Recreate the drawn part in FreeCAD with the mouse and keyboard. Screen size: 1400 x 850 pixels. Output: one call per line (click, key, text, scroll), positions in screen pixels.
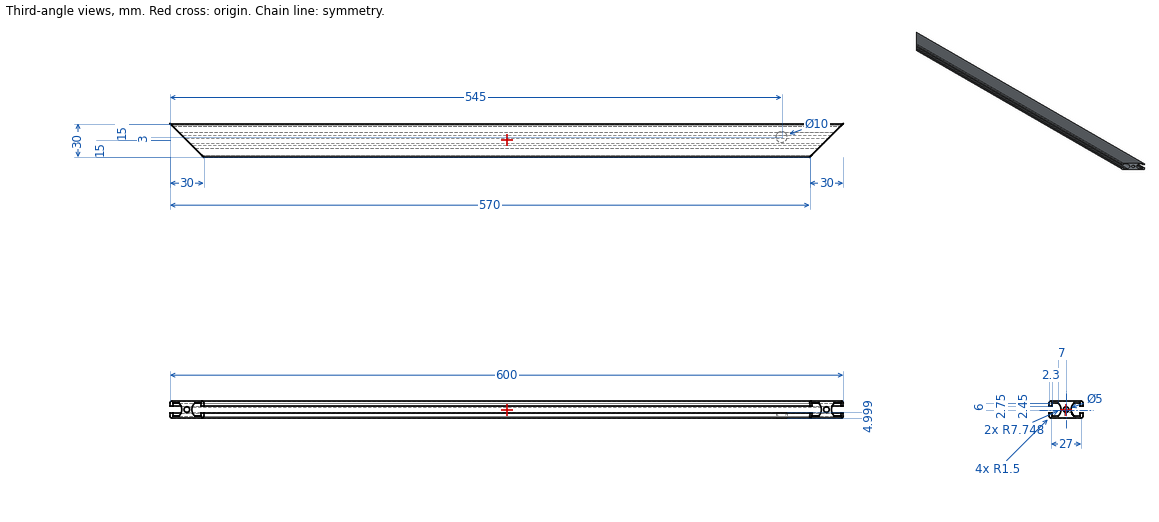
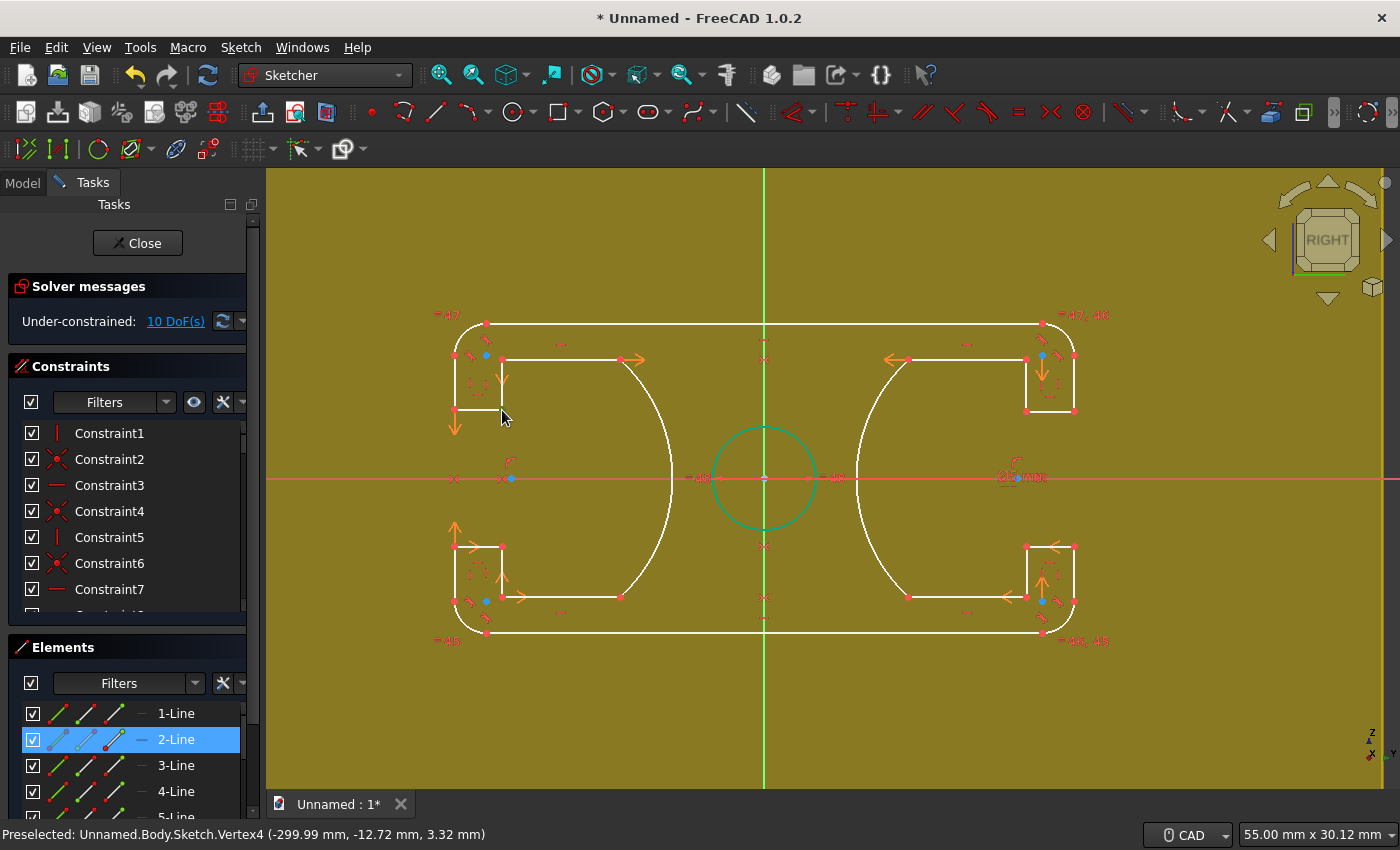
click(1026, 412)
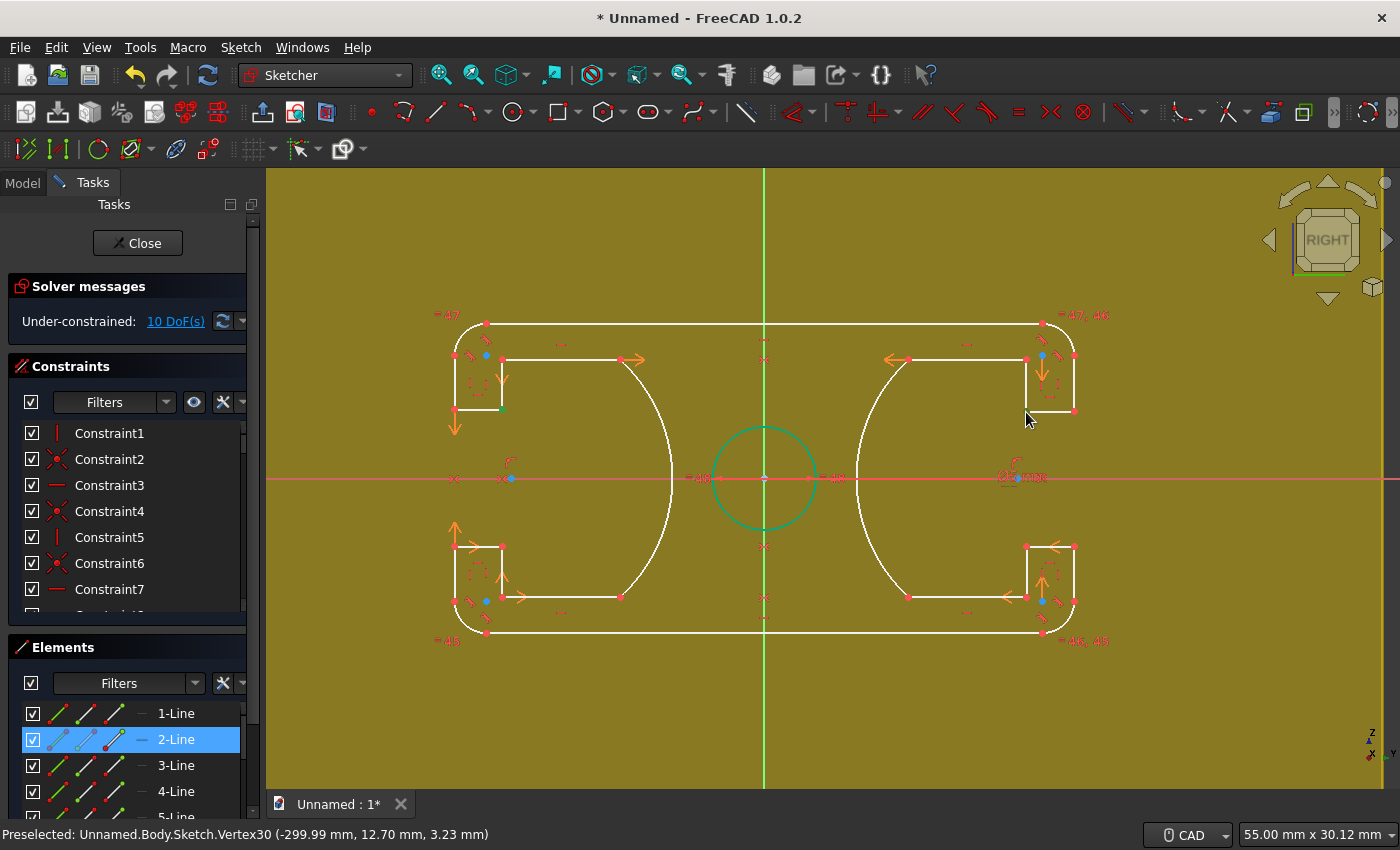
click(764, 721)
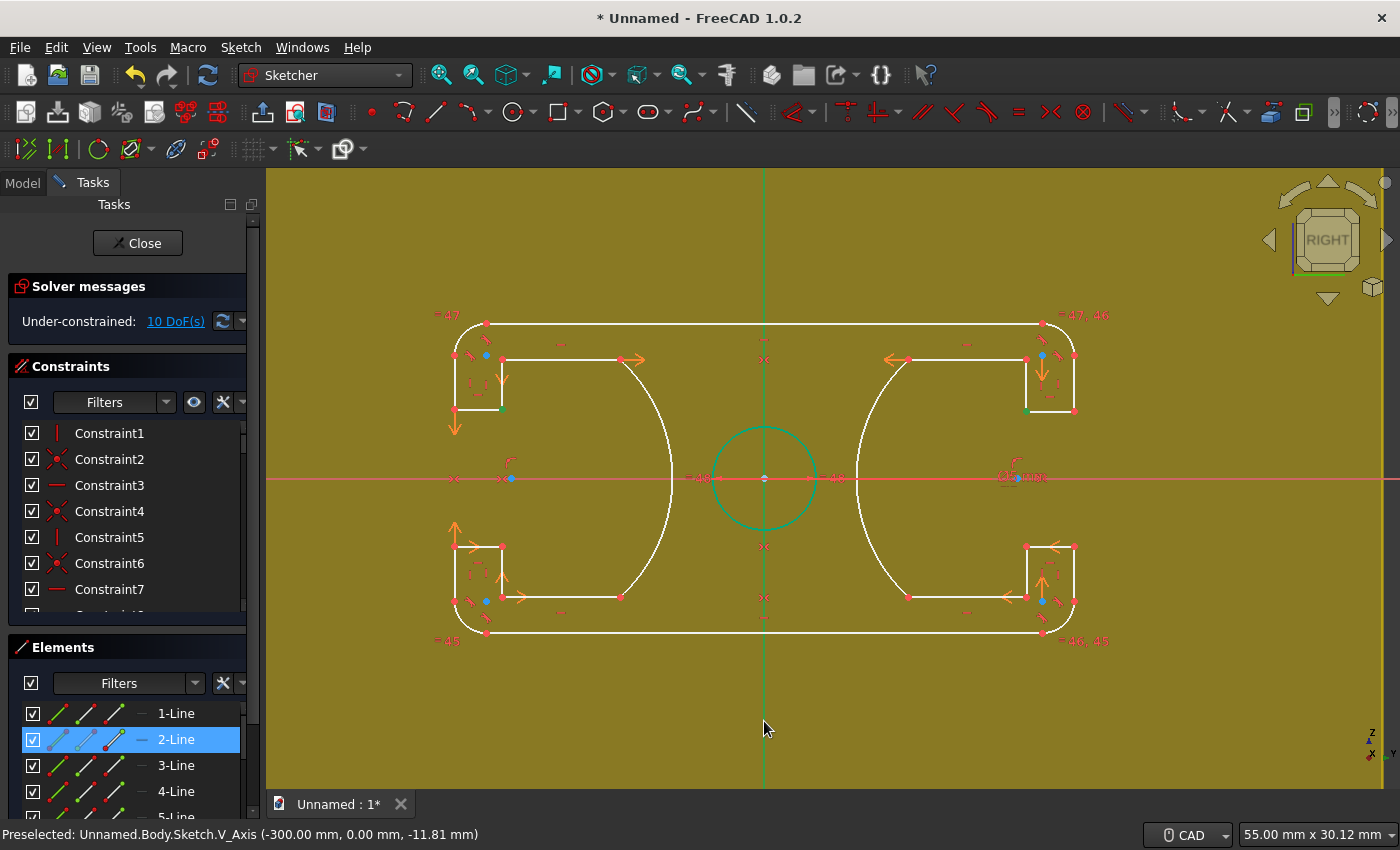
click(1052, 112)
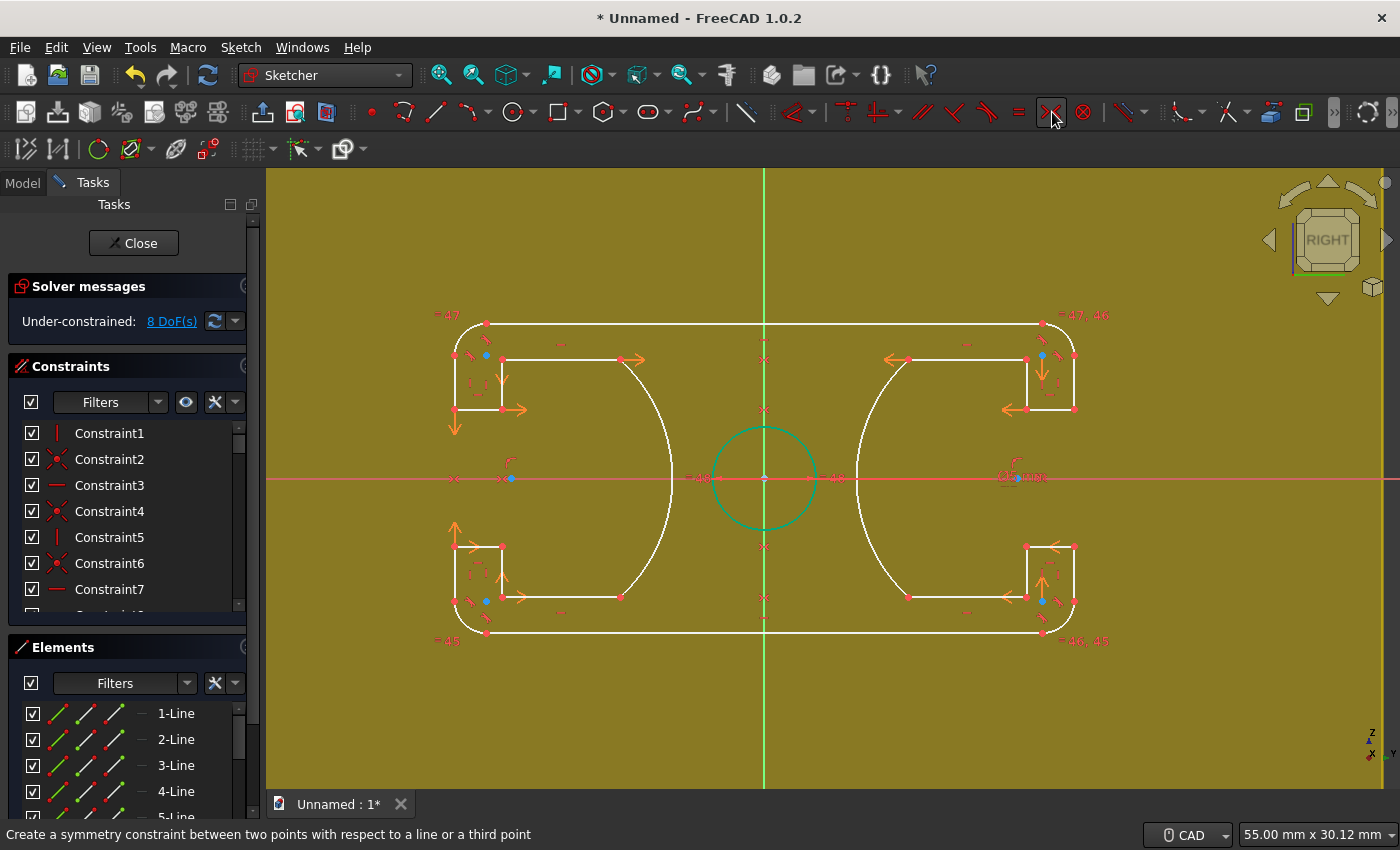
click(792, 112)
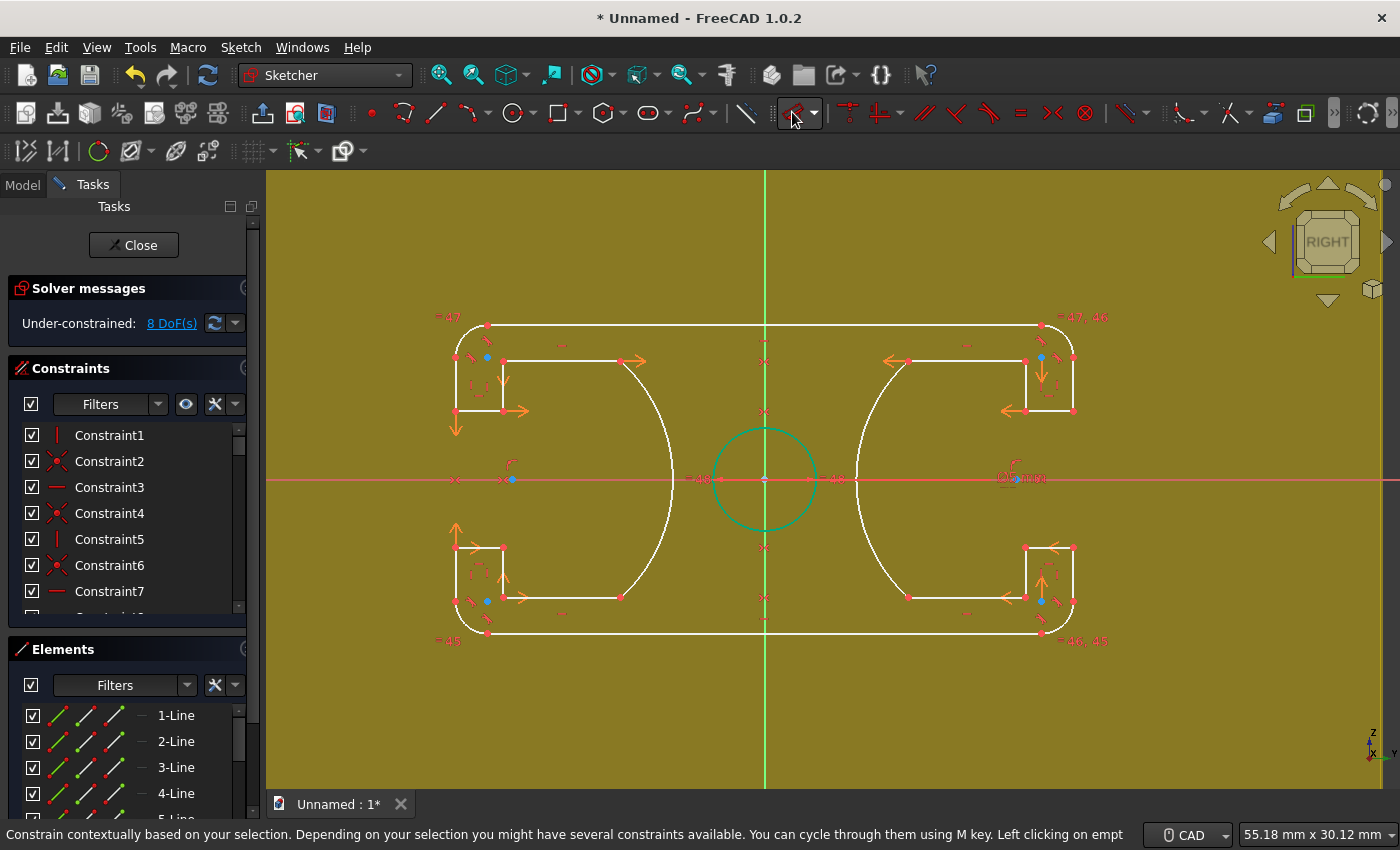
click(664, 532)
click(694, 542)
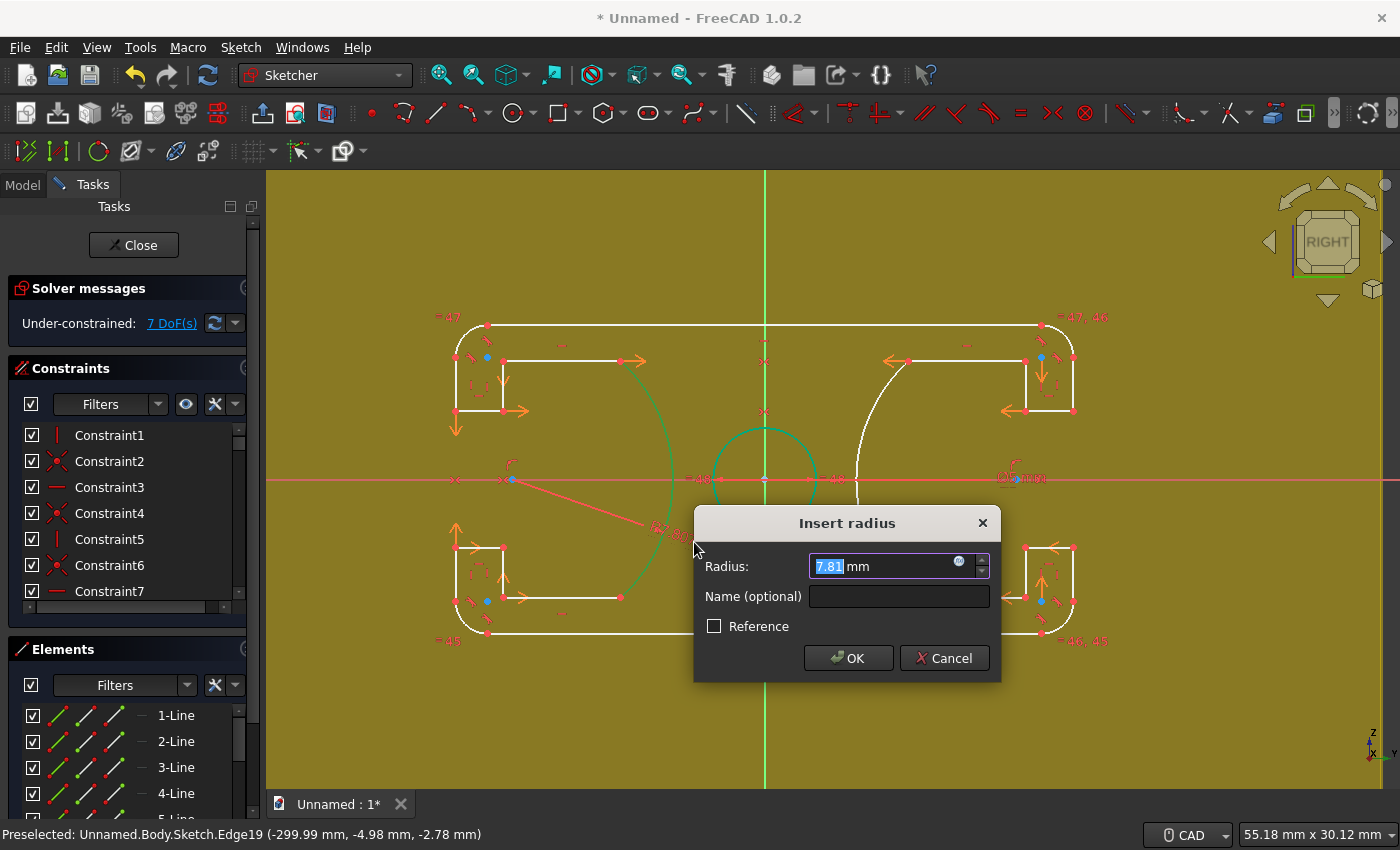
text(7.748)
key(Return)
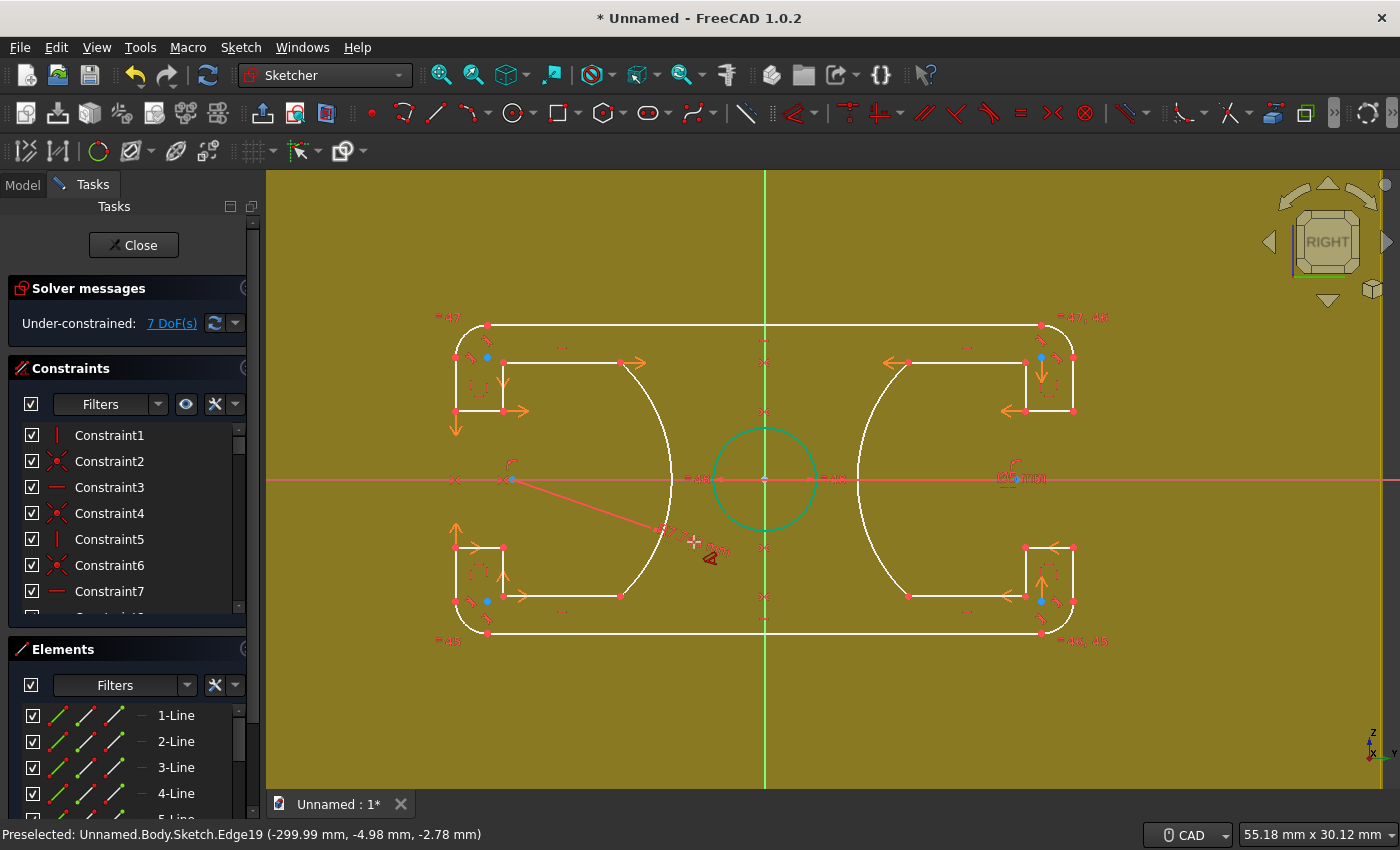
scroll(459, 616, up, 2)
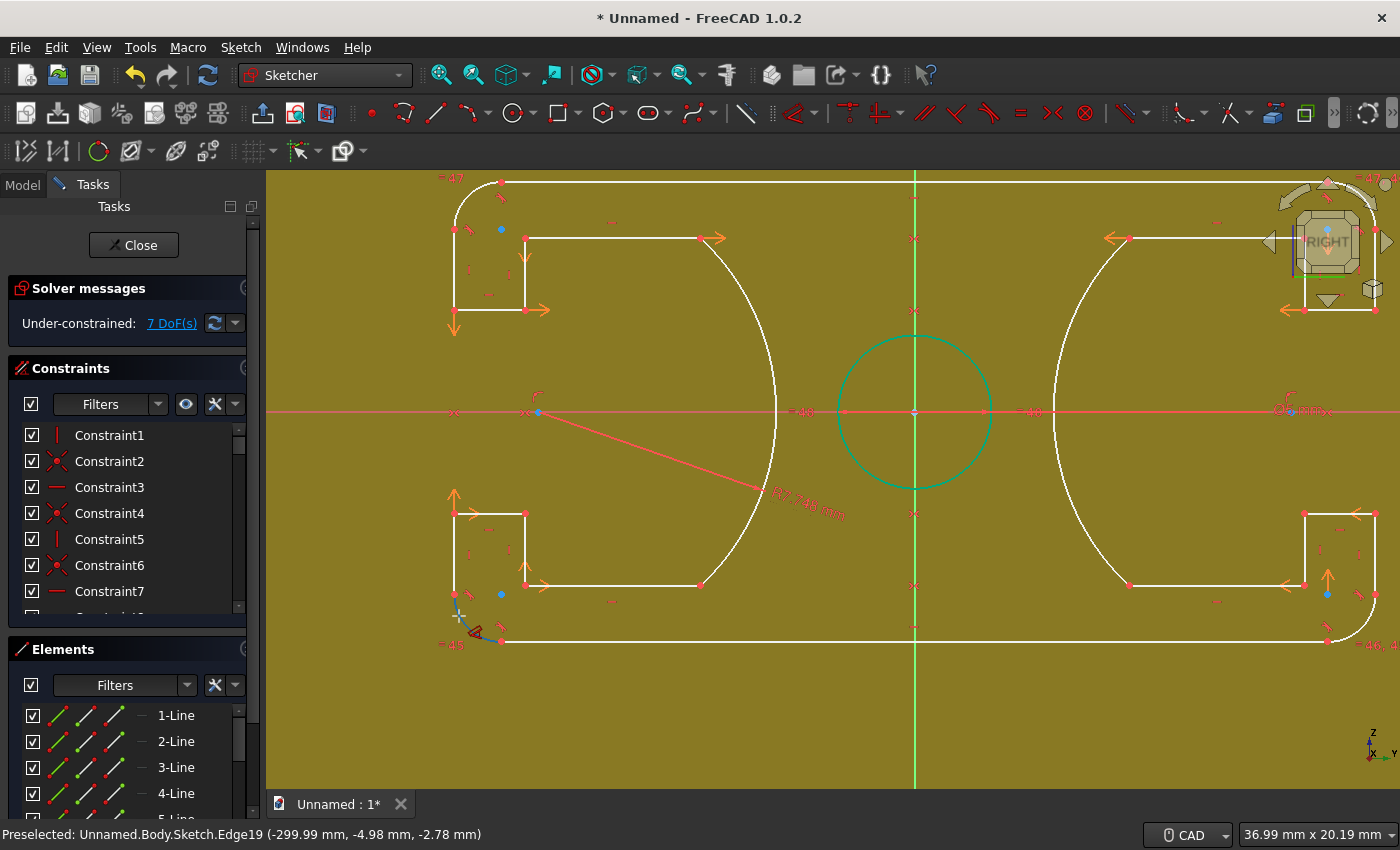
click(460, 616)
click(432, 631)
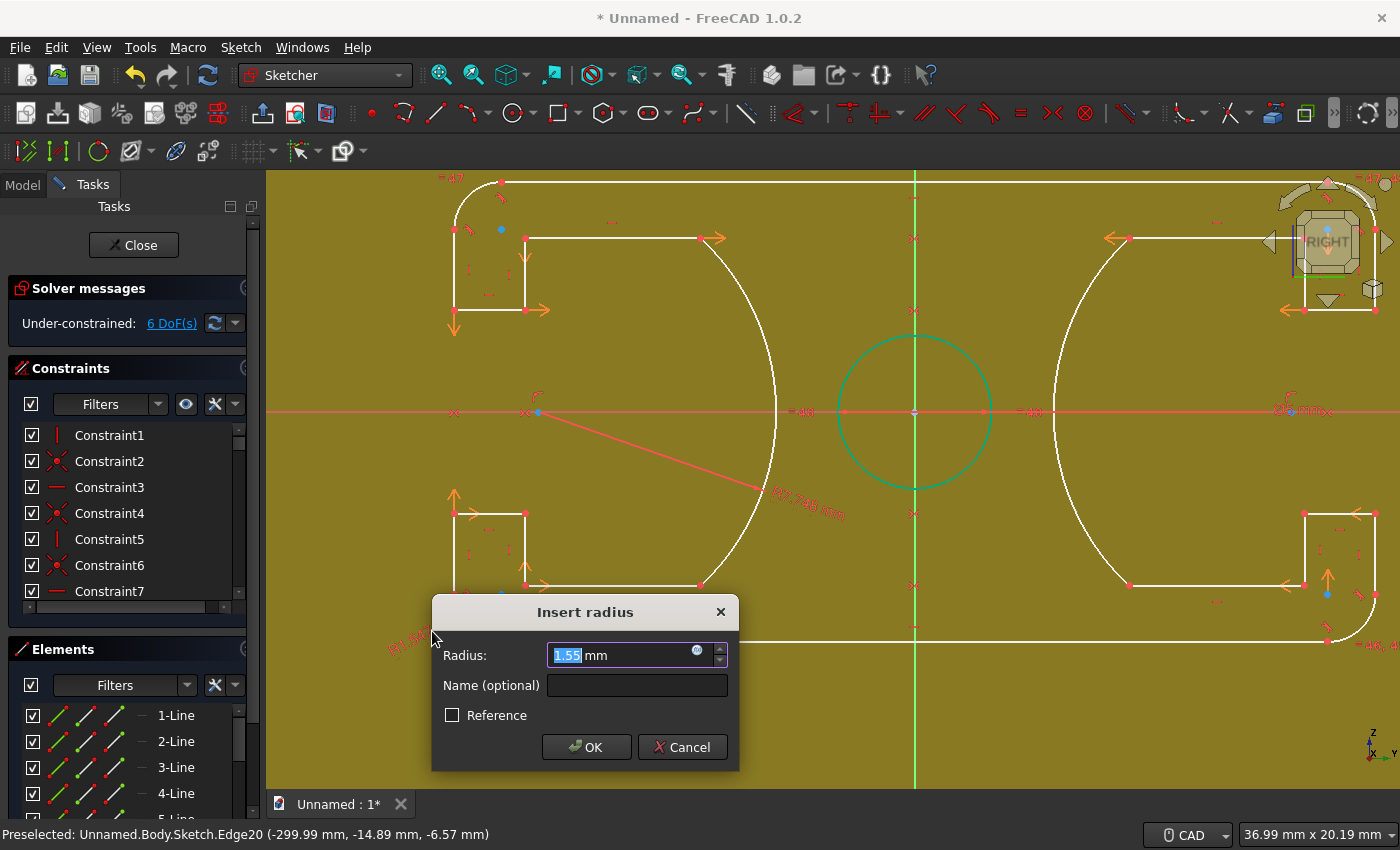
text(1.5)
key(Return)